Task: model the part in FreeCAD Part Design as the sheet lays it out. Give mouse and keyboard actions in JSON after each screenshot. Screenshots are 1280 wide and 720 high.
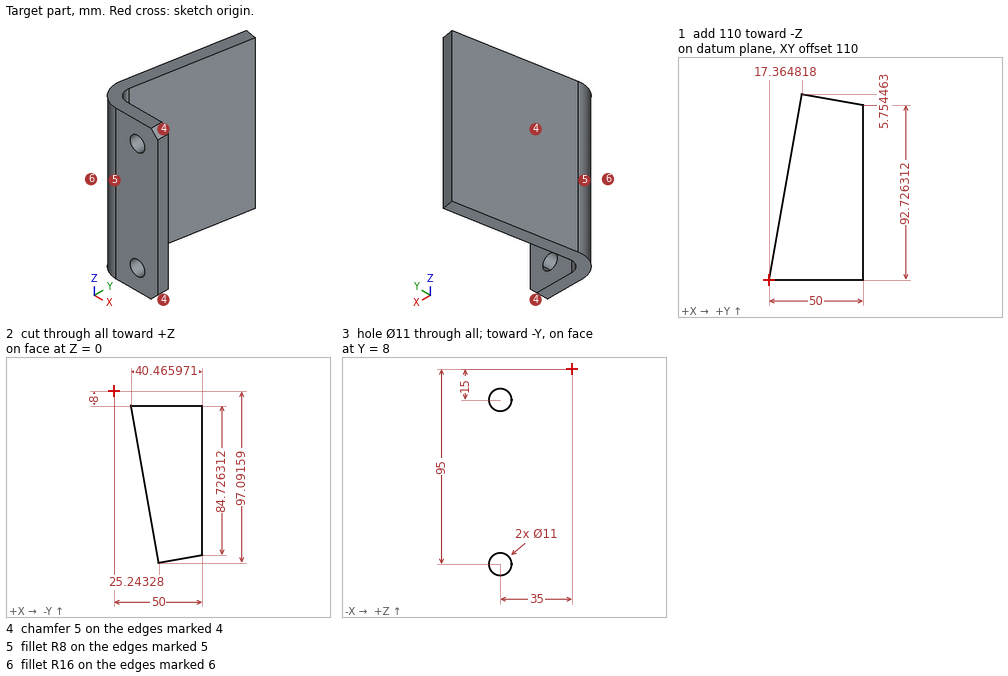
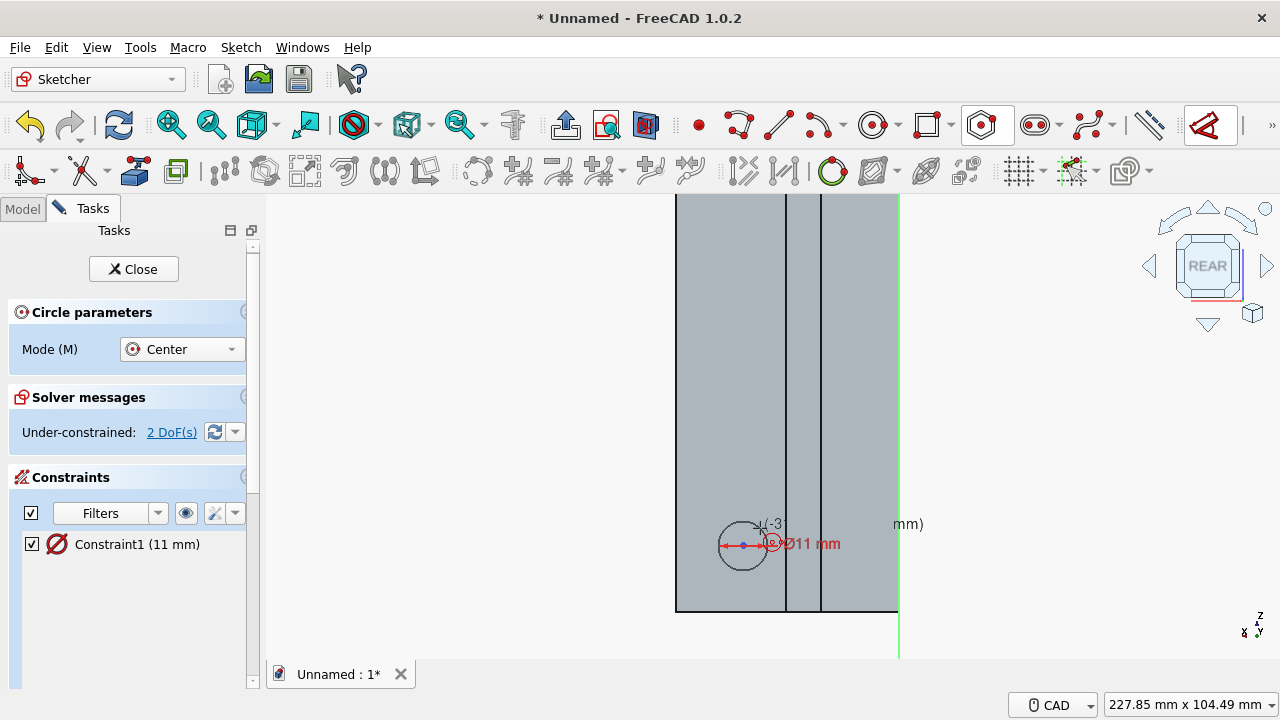
{"action": "scroll", "coordinate": [493, 590], "scroll_direction": "down", "scroll_amount": 2}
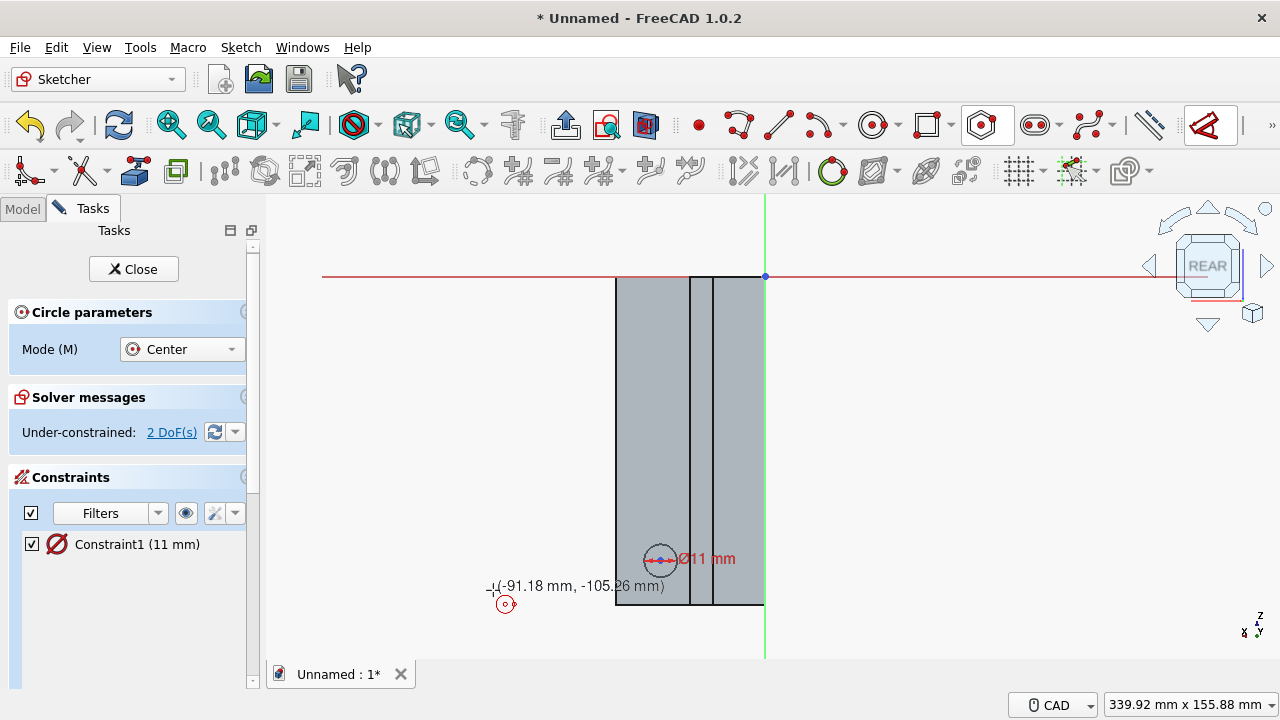
{"action": "scroll", "coordinate": [661, 322], "scroll_direction": "up", "scroll_amount": 2}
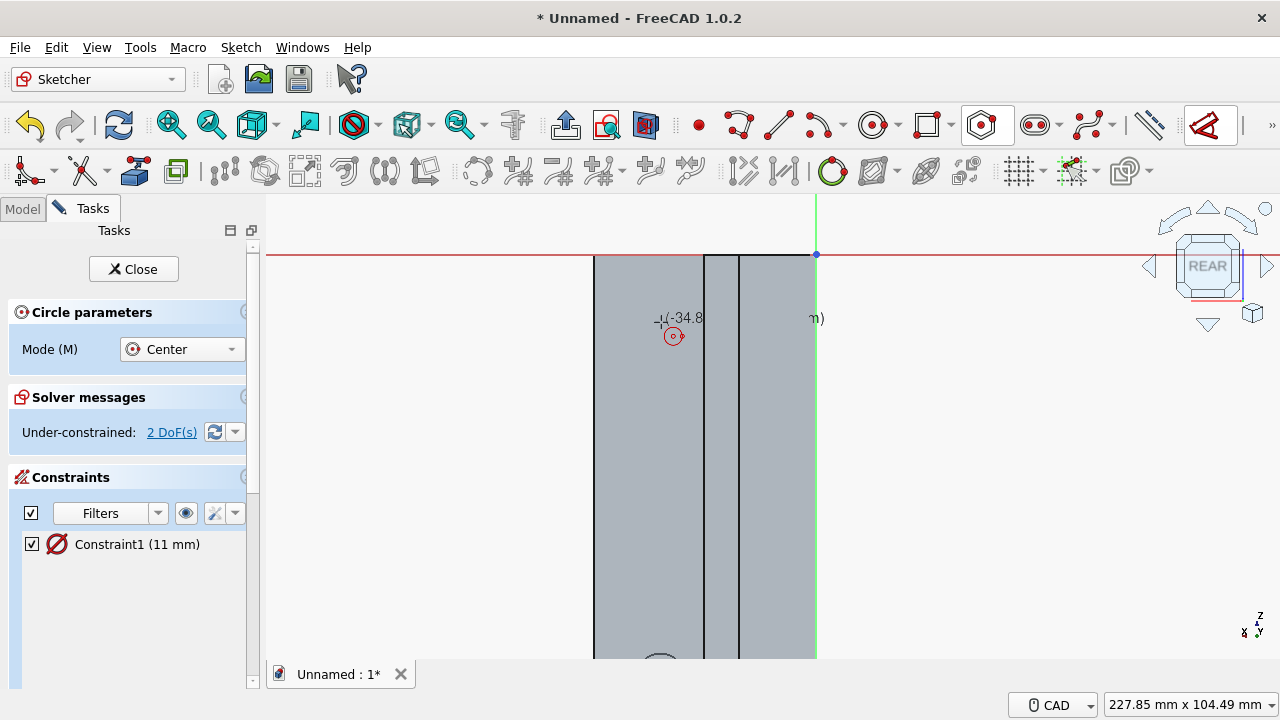
{"action": "left_click", "coordinate": [660, 321]}
{"action": "mouse_move", "coordinate": [678, 304]}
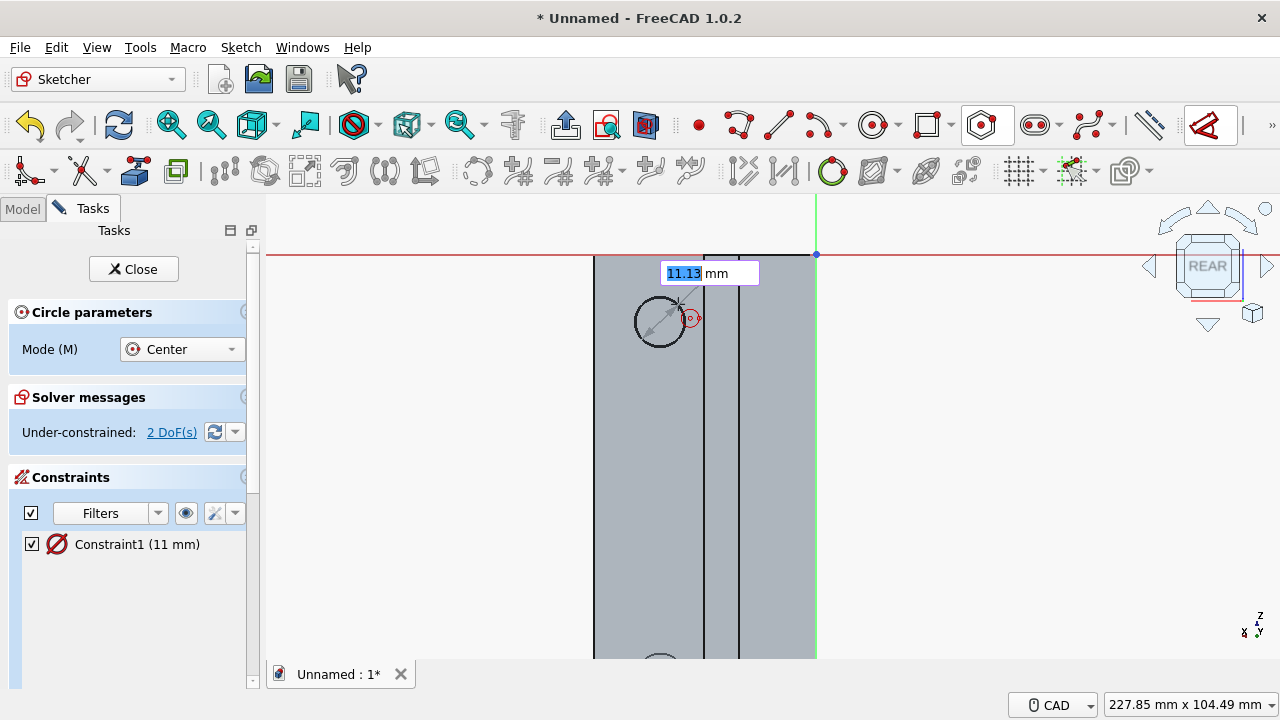
{"action": "type", "text": "11"}
{"action": "key", "text": "Return"}
{"action": "key", "text": "Escape"}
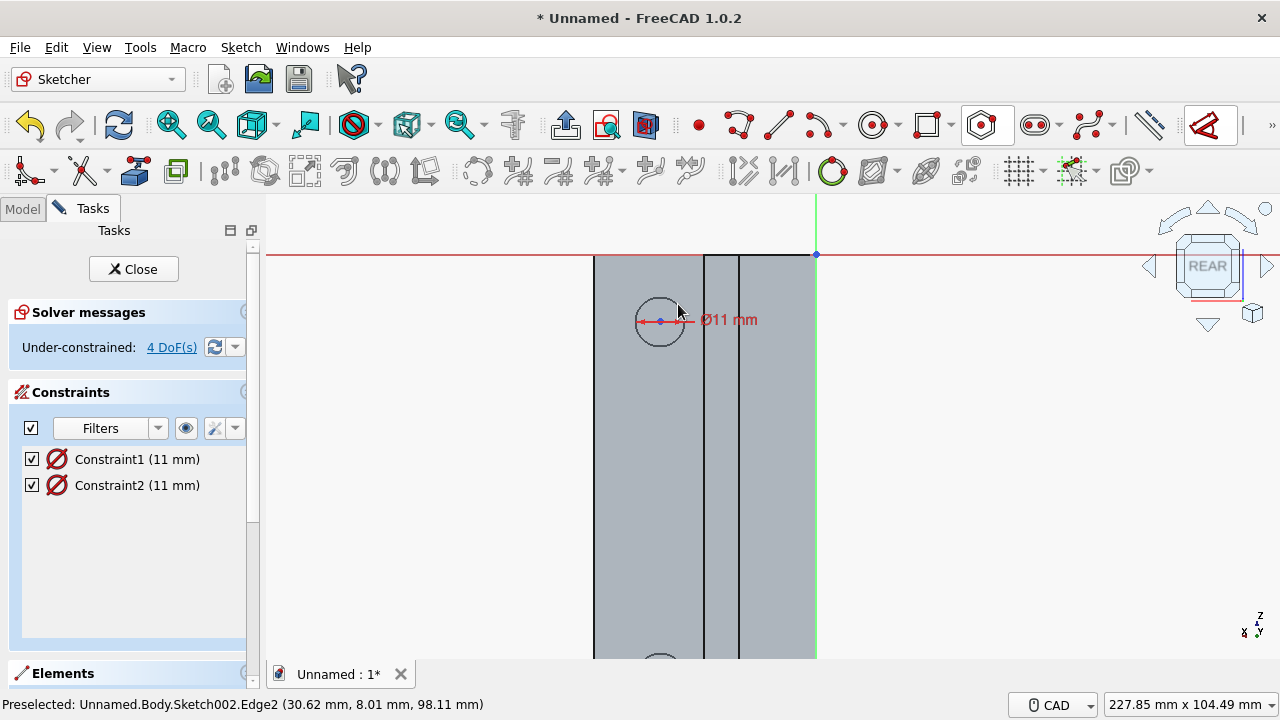
{"action": "scroll", "coordinate": [661, 321], "scroll_direction": "down", "scroll_amount": 2}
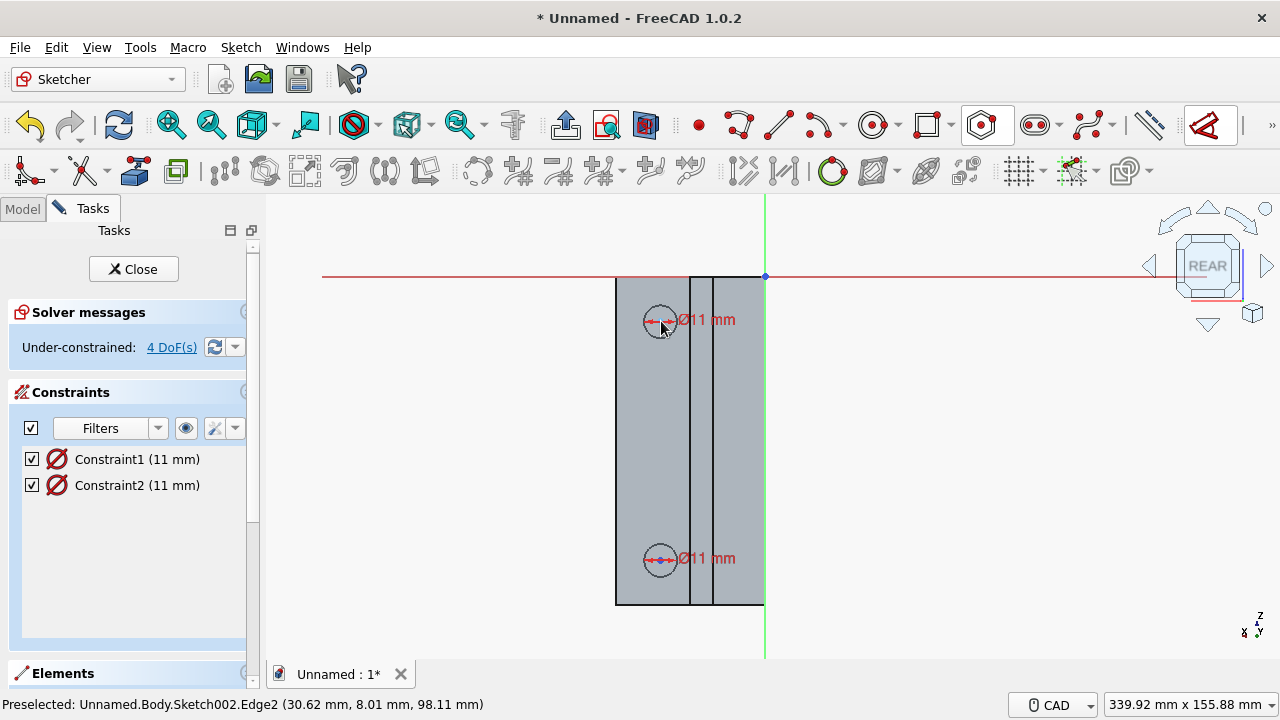
{"action": "left_click", "coordinate": [661, 560]}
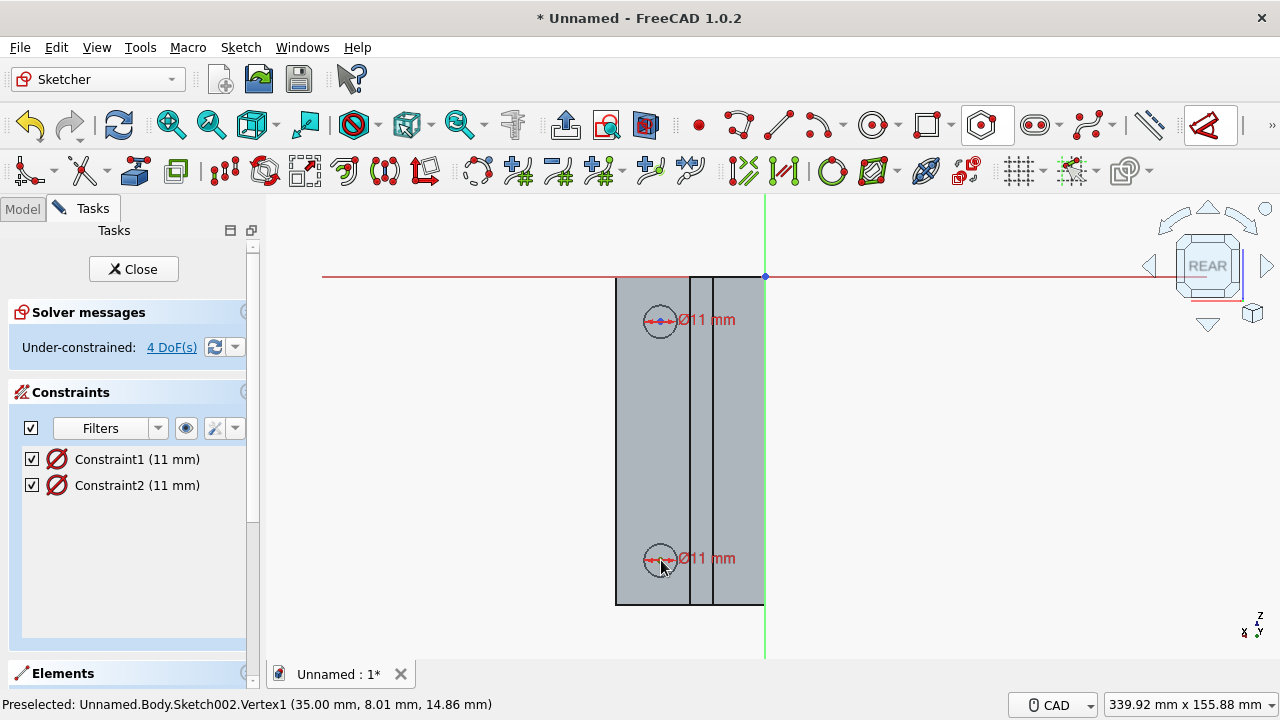
{"action": "left_click", "coordinate": [660, 322]}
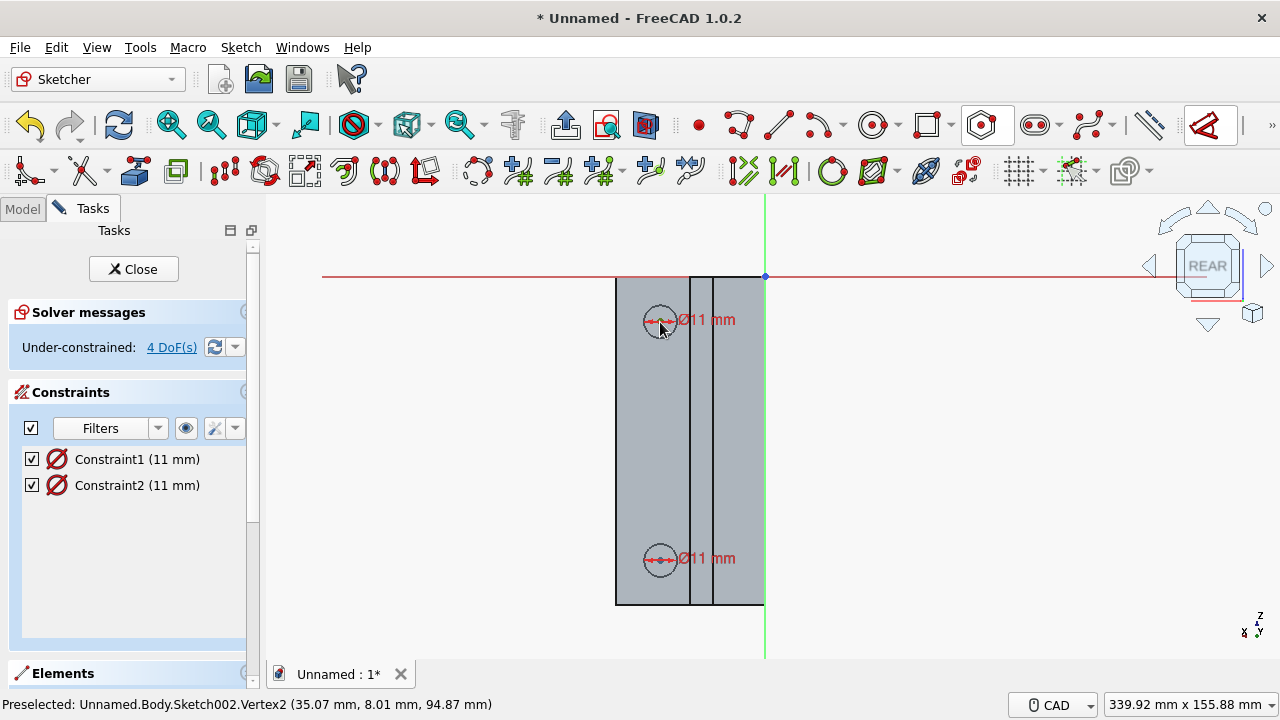
{"action": "key", "text": "v"}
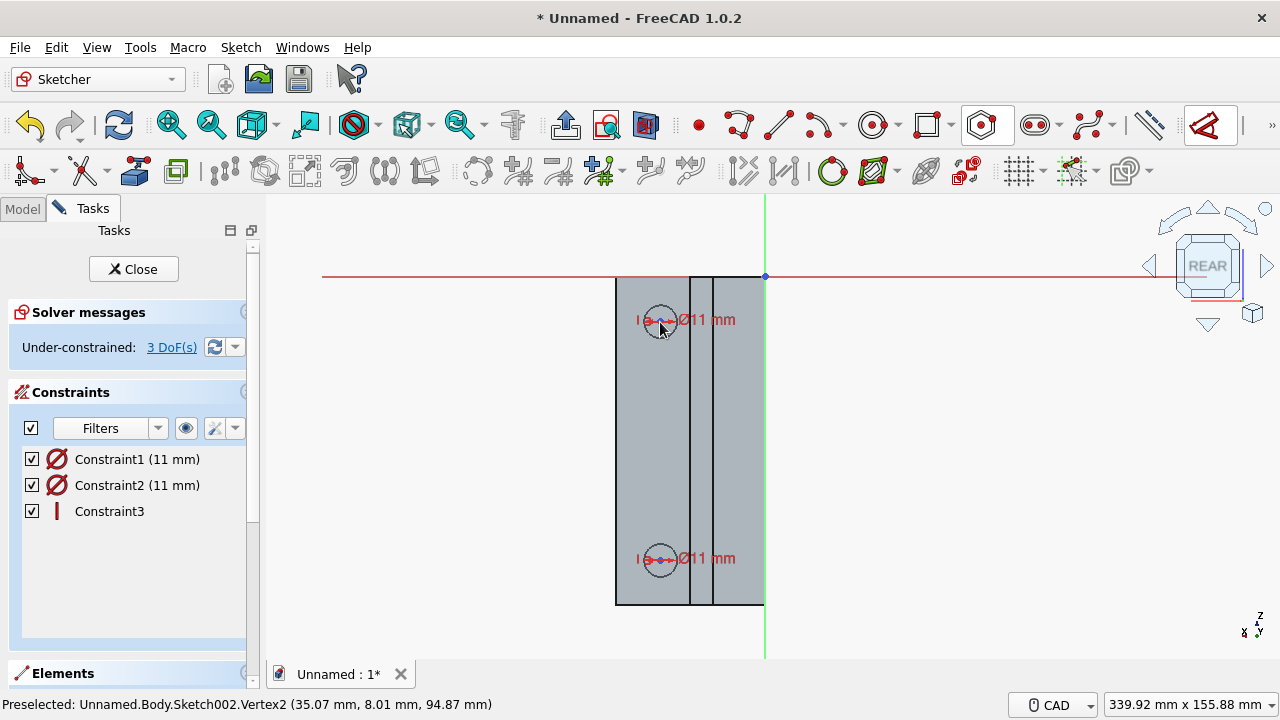
{"action": "left_click", "coordinate": [661, 560]}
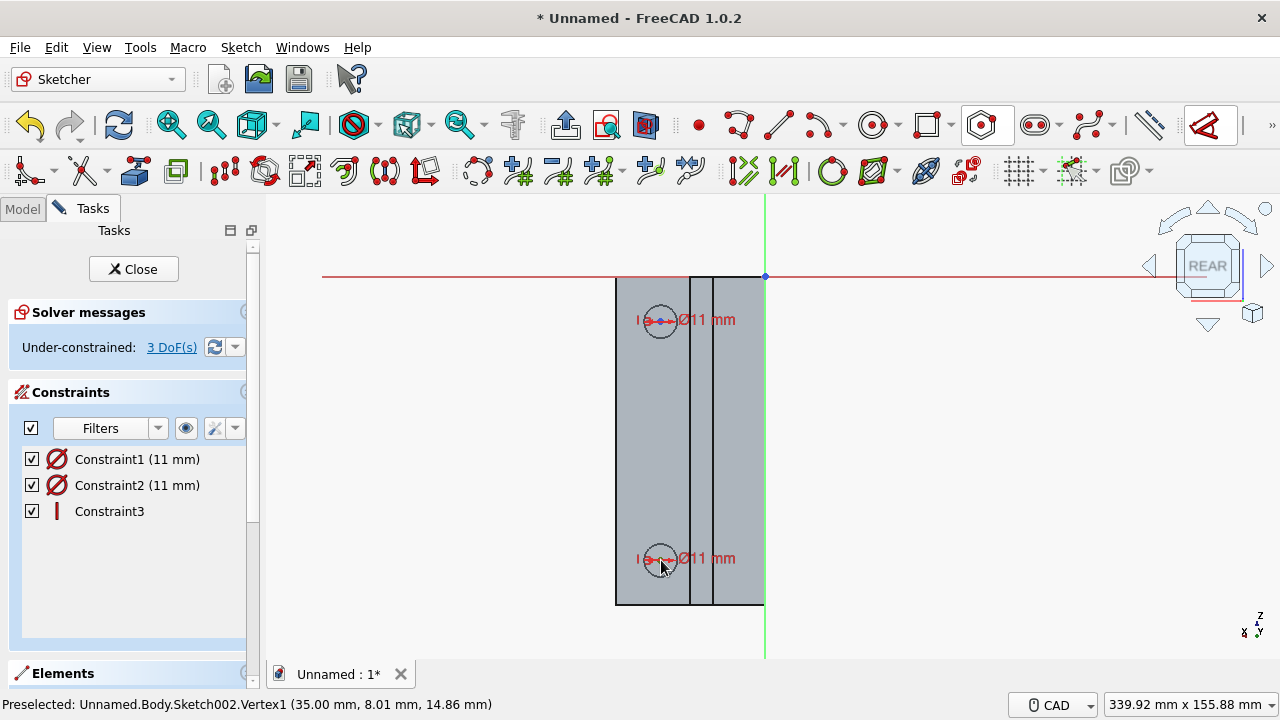
{"action": "key", "text": "l"}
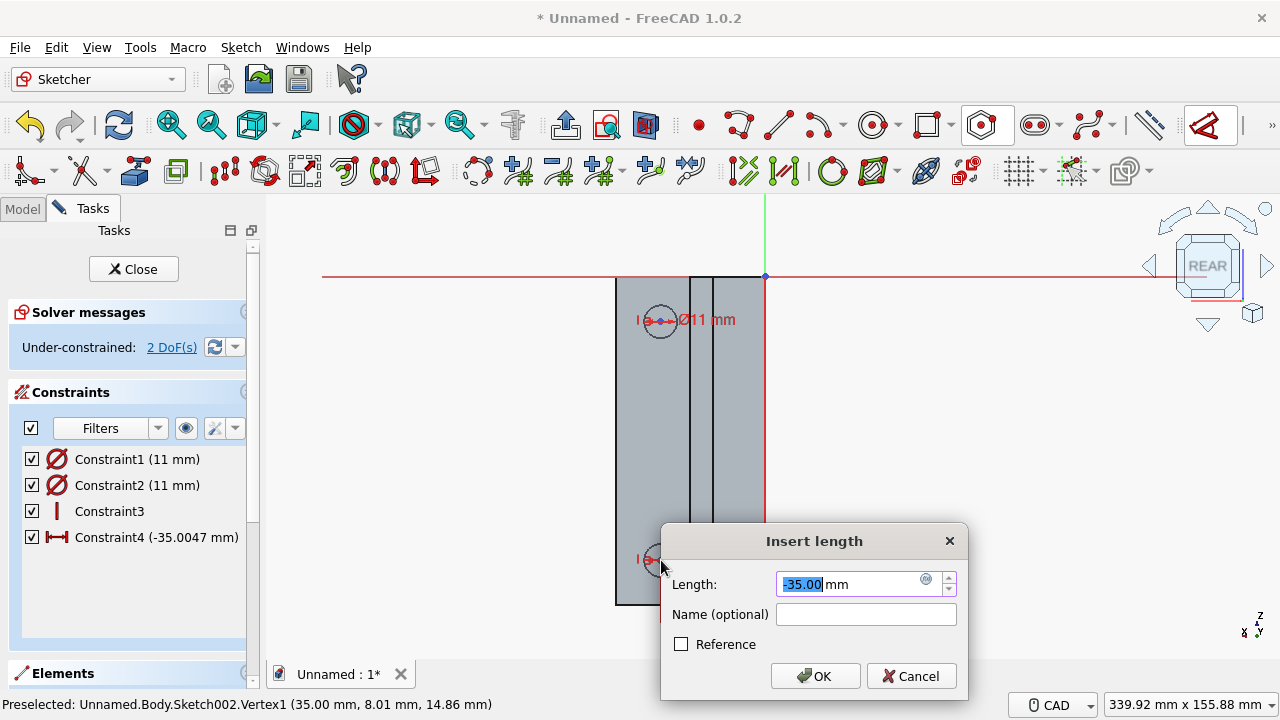
{"action": "type", "text": "-35"}
{"action": "key", "text": "Return"}